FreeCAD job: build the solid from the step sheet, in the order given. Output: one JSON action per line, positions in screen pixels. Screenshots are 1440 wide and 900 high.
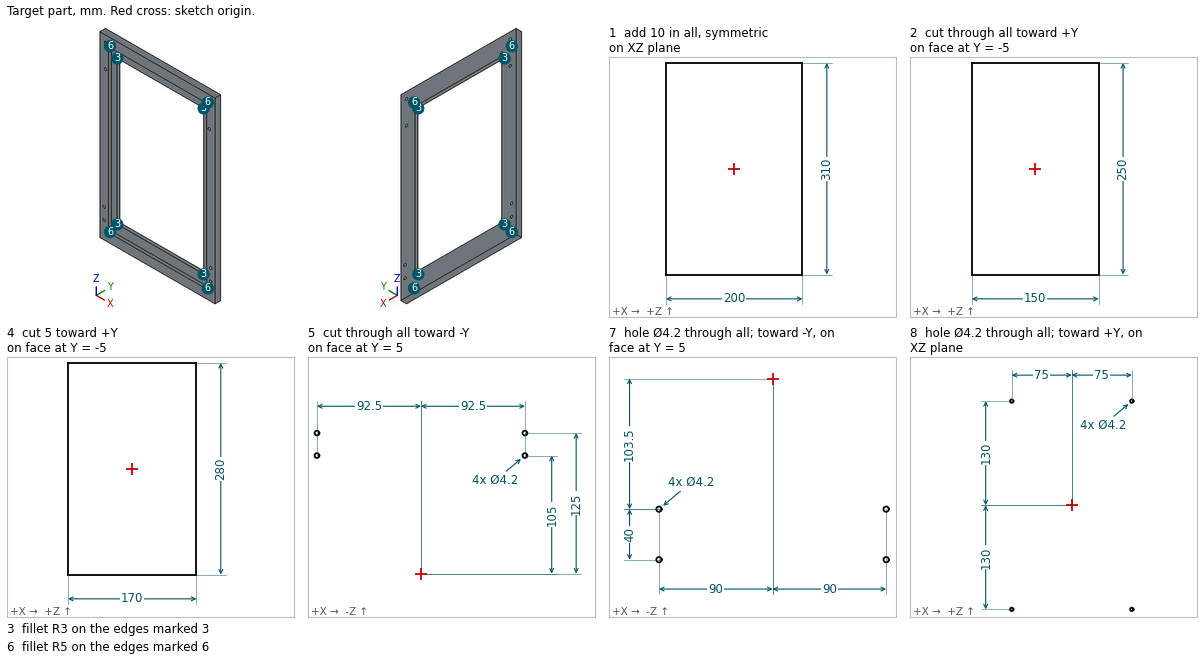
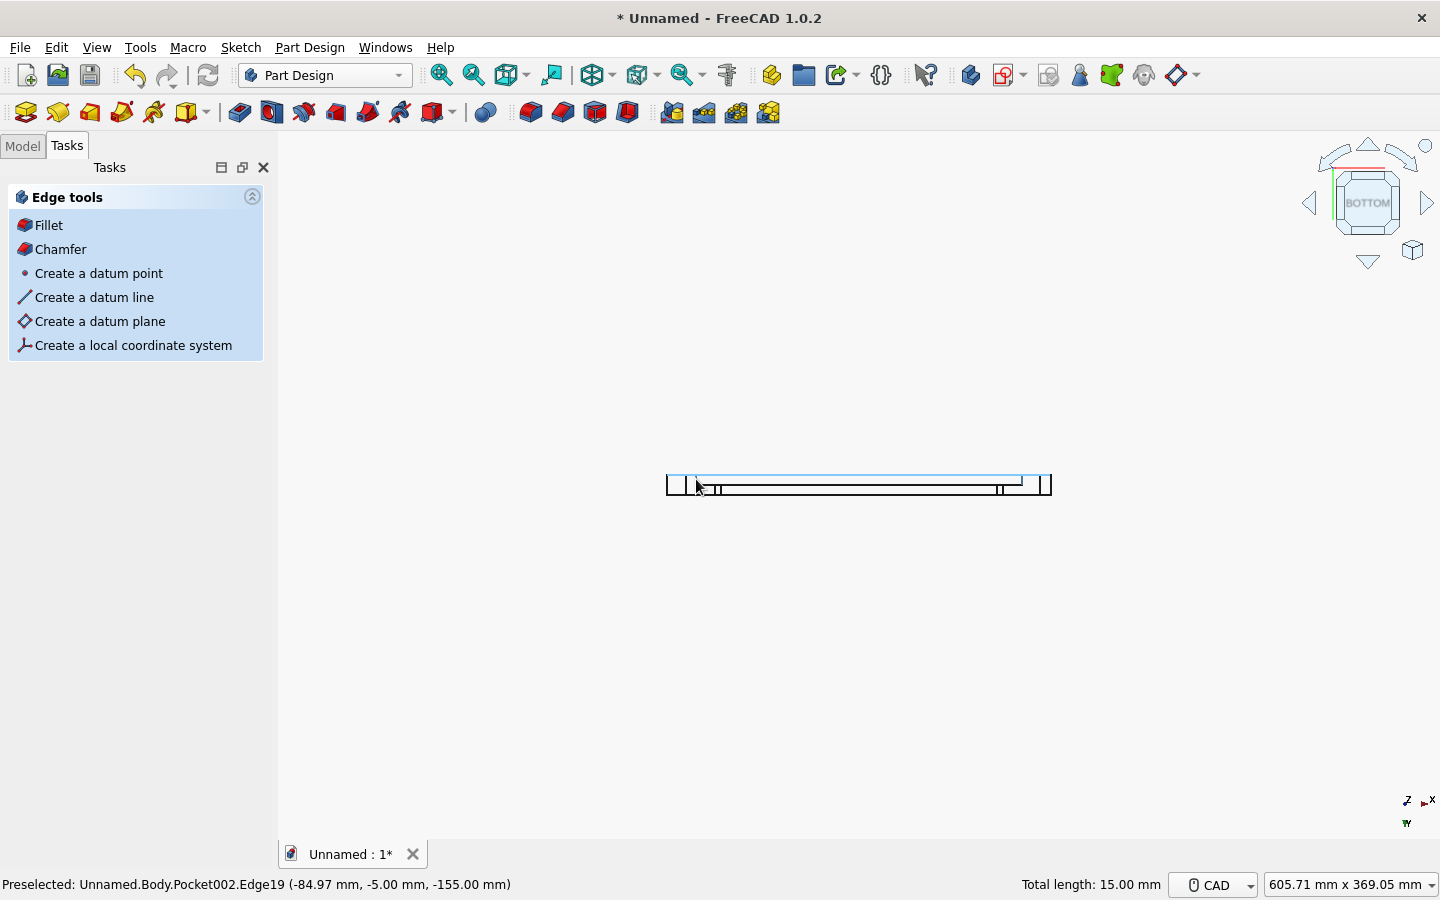
{"action": "key", "text": "4"}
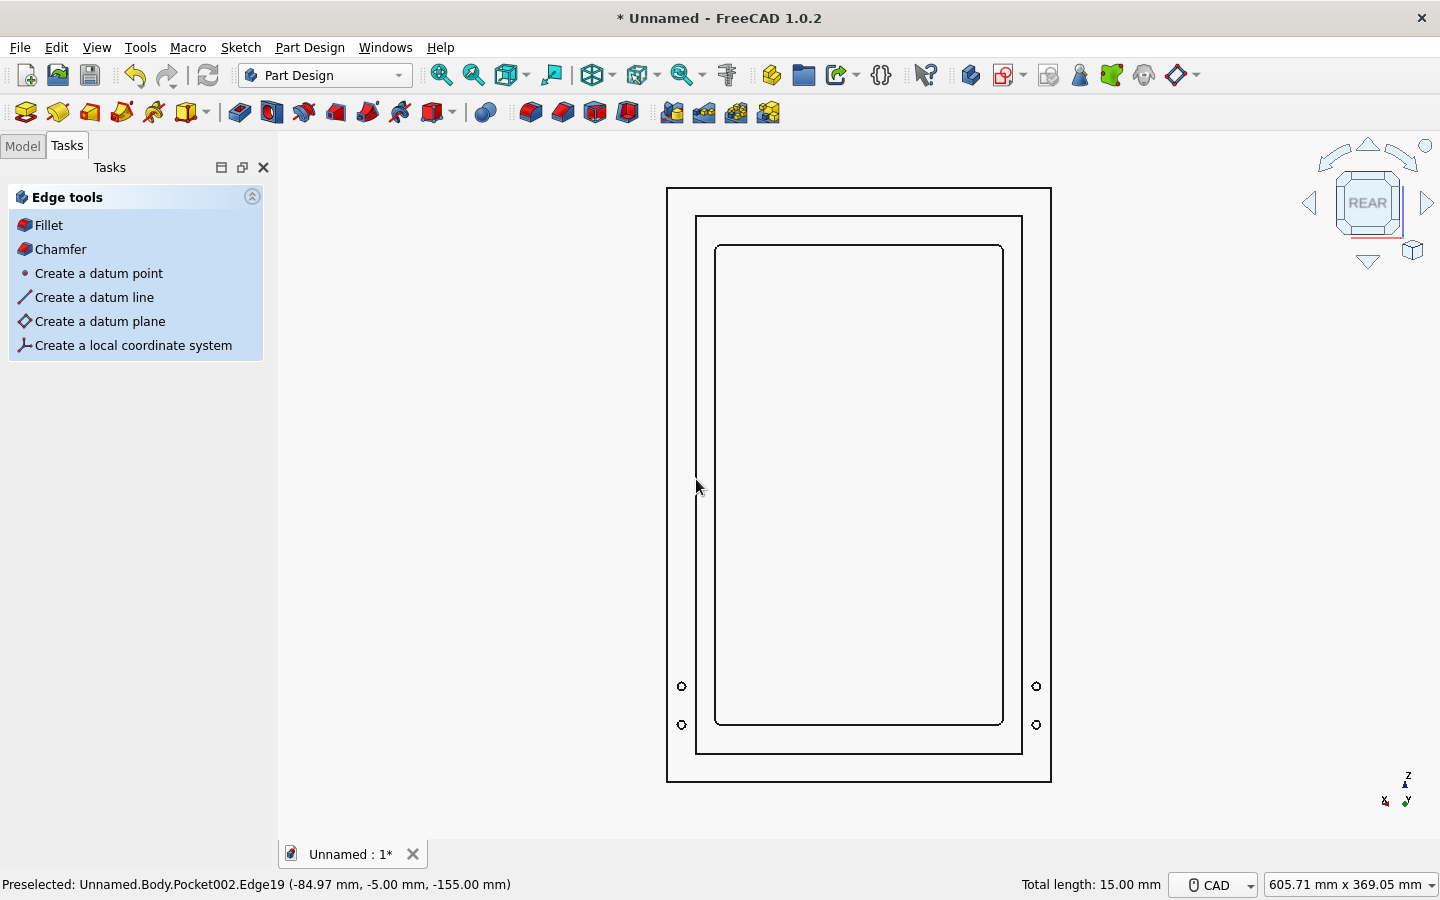
{"action": "scroll", "coordinate": [1022, 215], "scroll_direction": "up", "scroll_amount": 8}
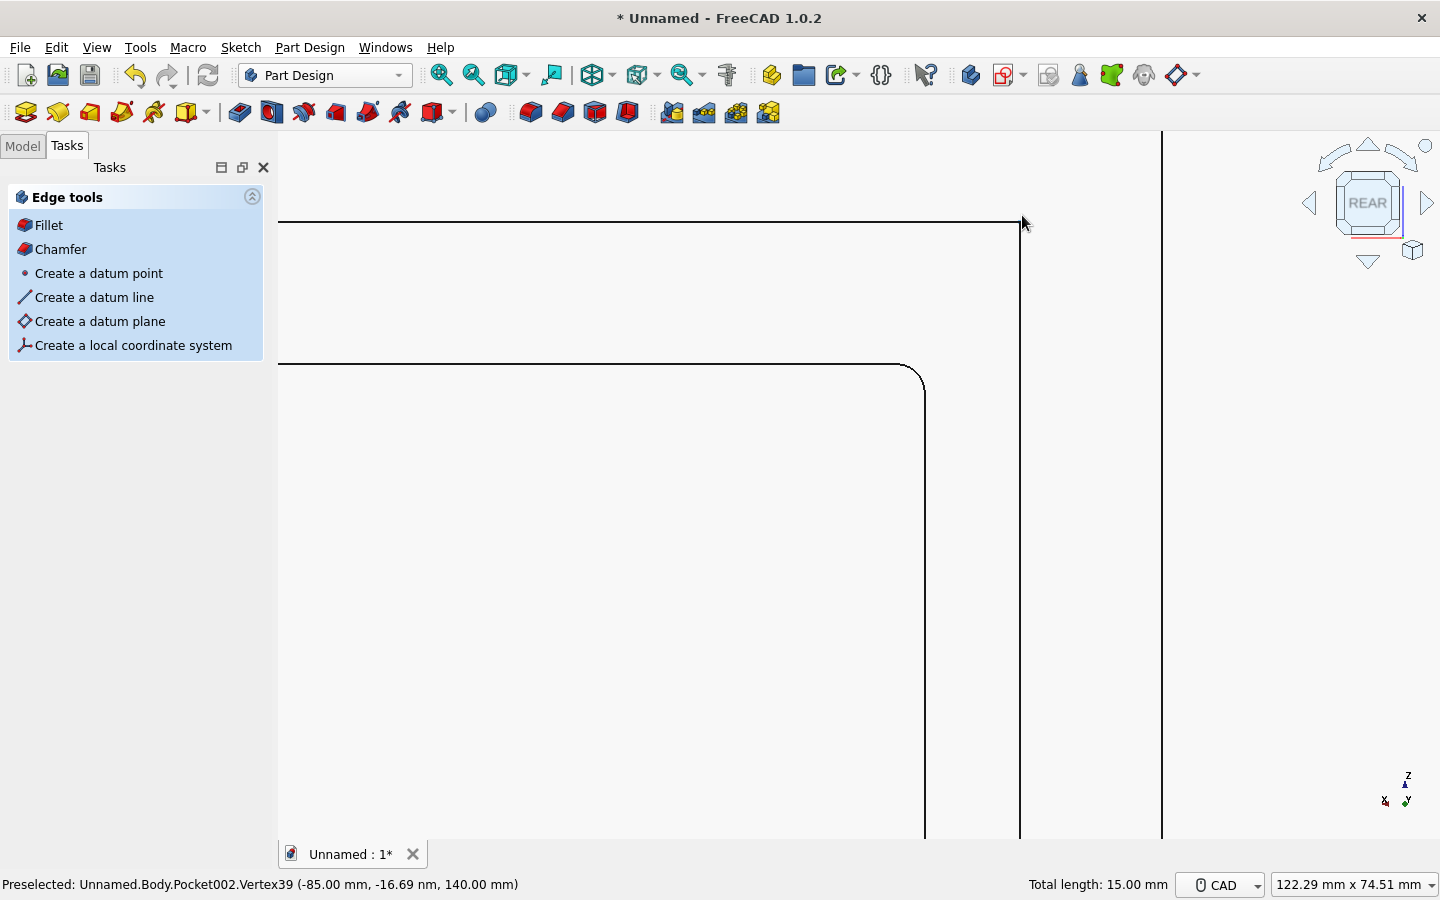
{"action": "left_click", "coordinate": [442, 76]}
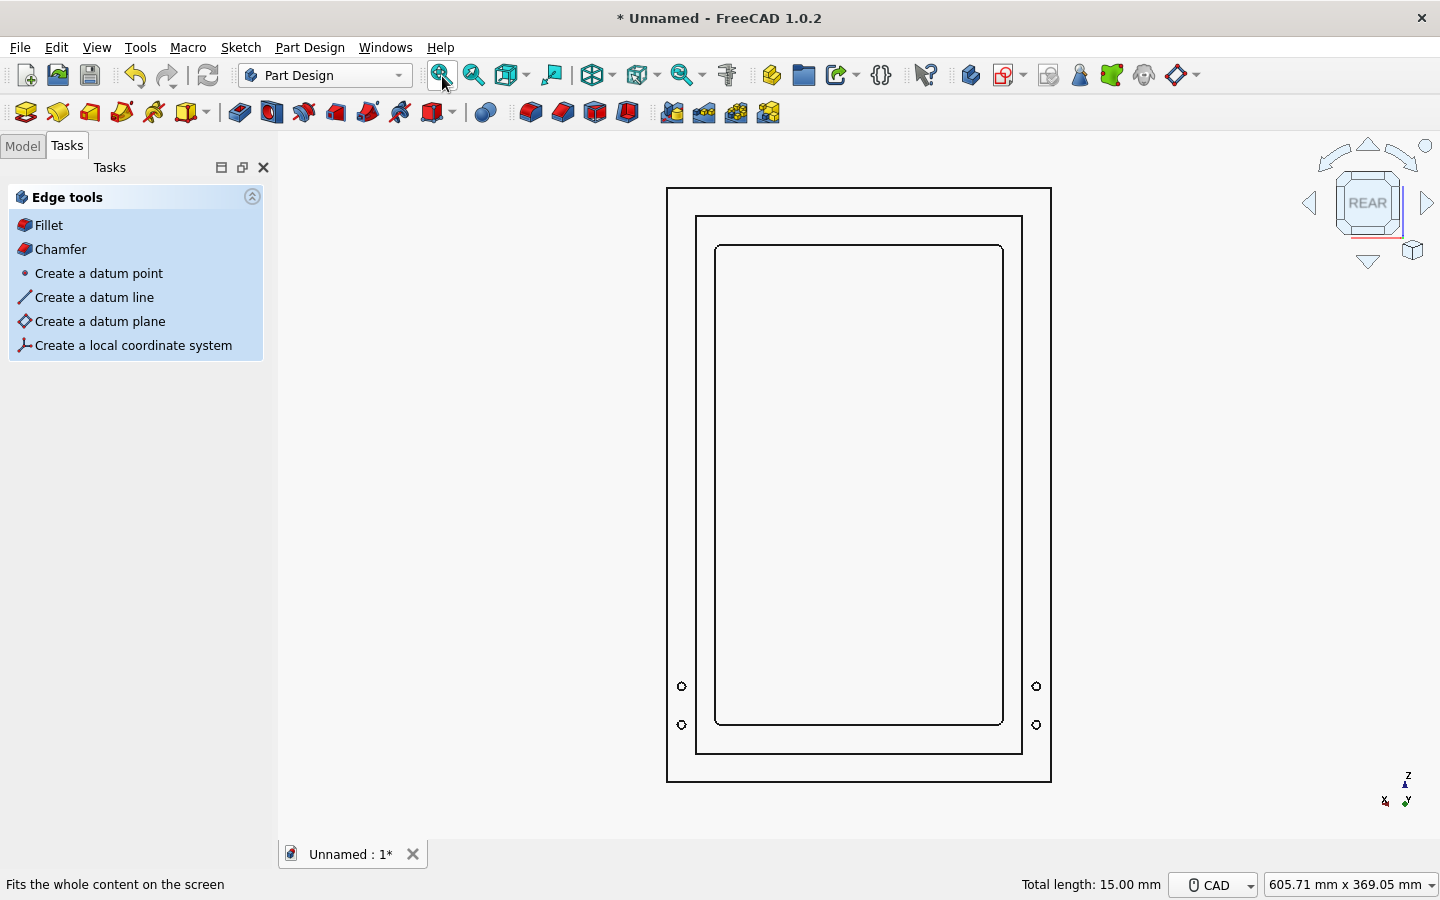
{"action": "key", "text": "6"}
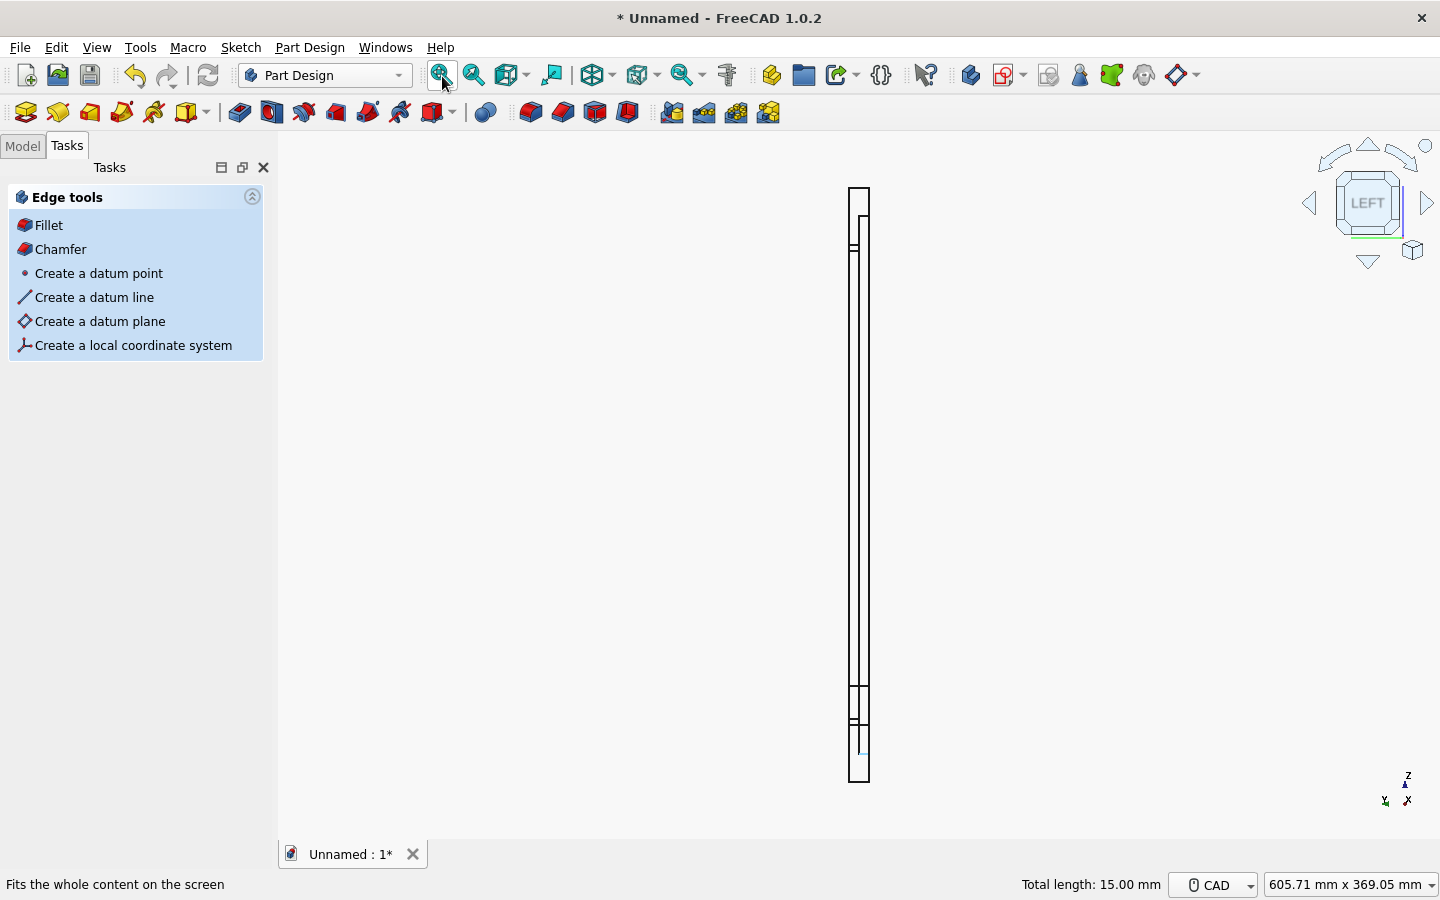
{"action": "scroll", "coordinate": [864, 215], "scroll_direction": "up", "scroll_amount": 8}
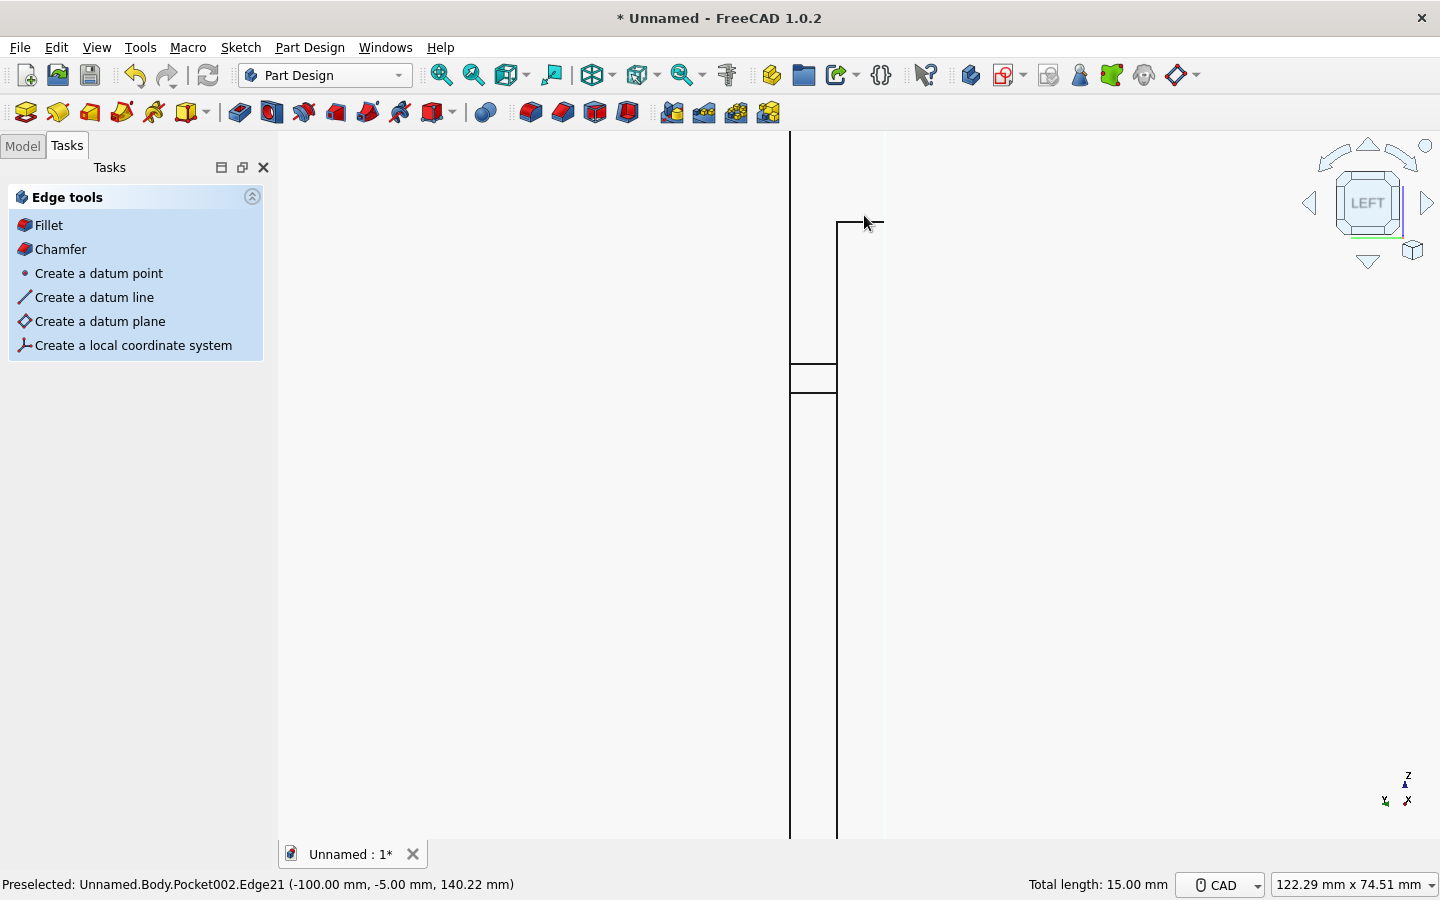
{"action": "left_click", "coordinate": [861, 221], "text": "ctrl"}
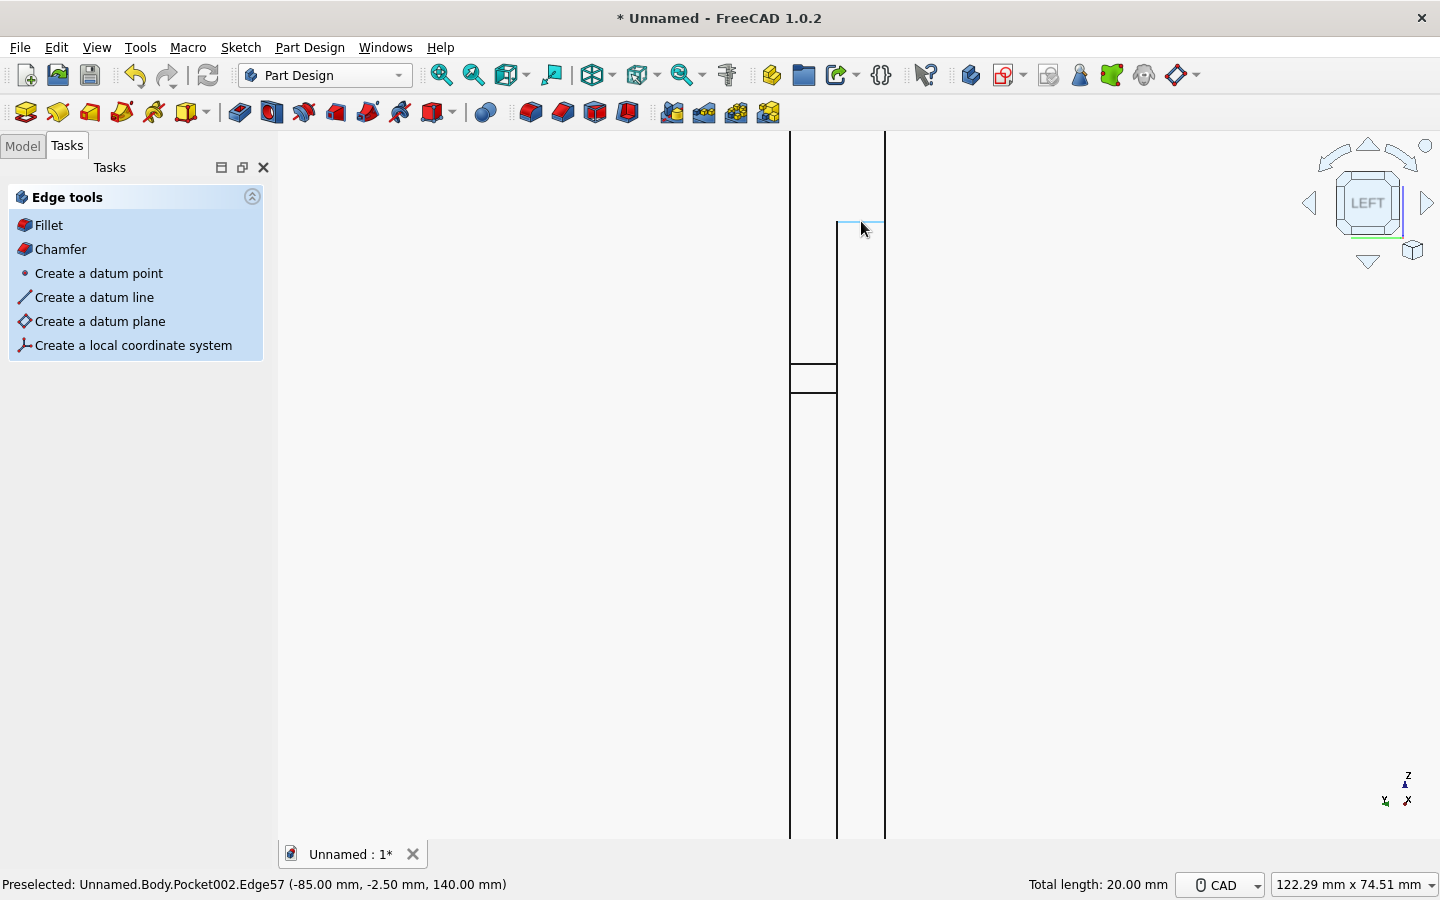
{"action": "key", "text": "v 1"}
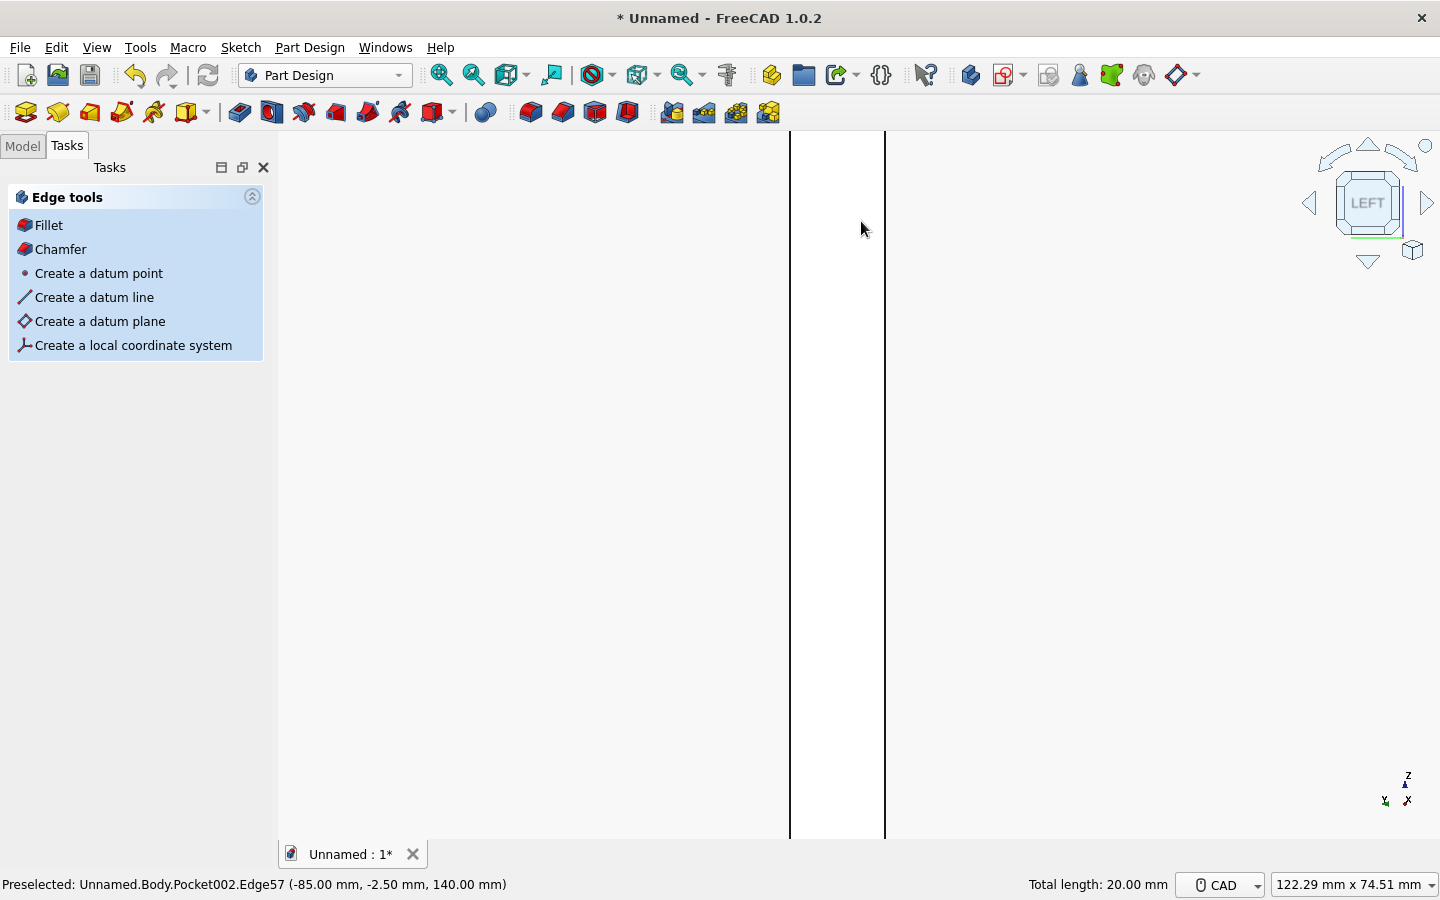
{"action": "left_click", "coordinate": [532, 112]}